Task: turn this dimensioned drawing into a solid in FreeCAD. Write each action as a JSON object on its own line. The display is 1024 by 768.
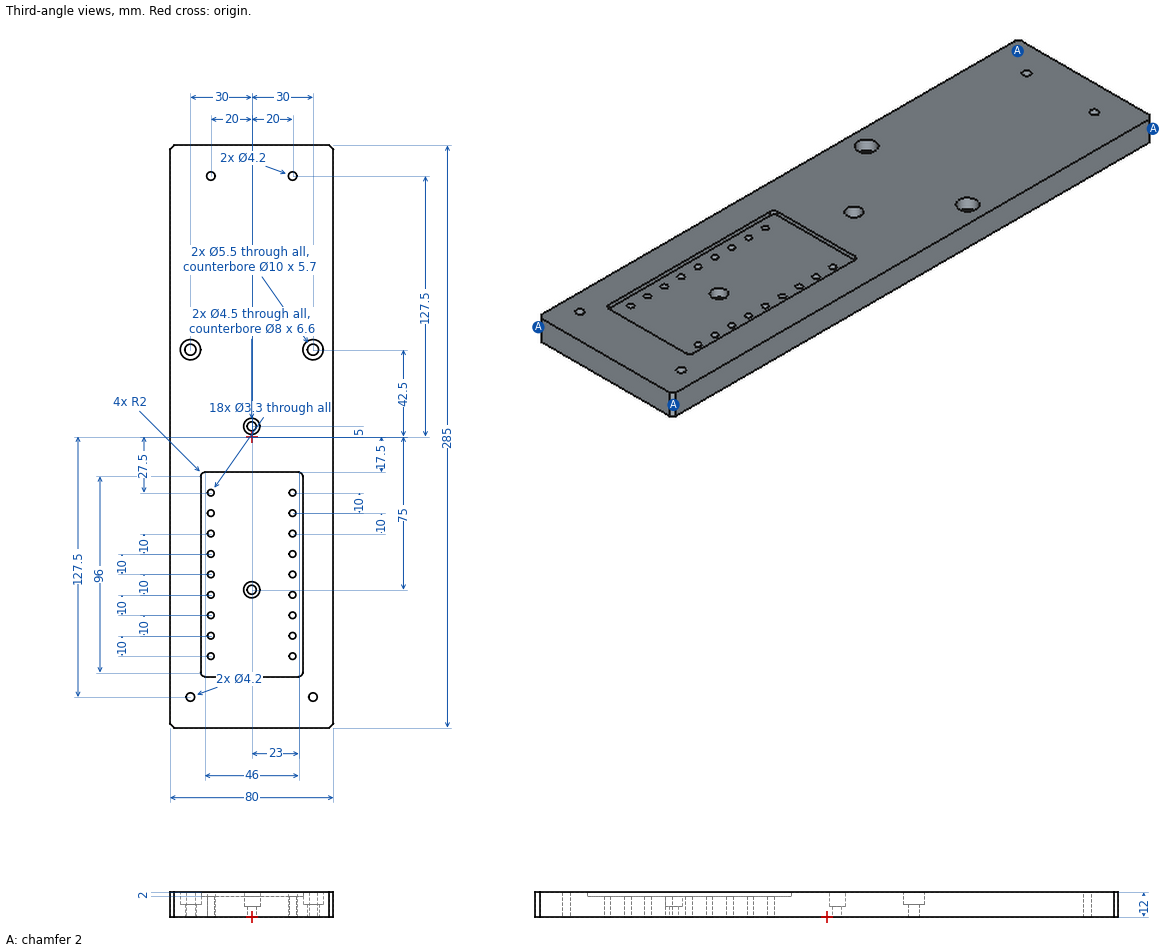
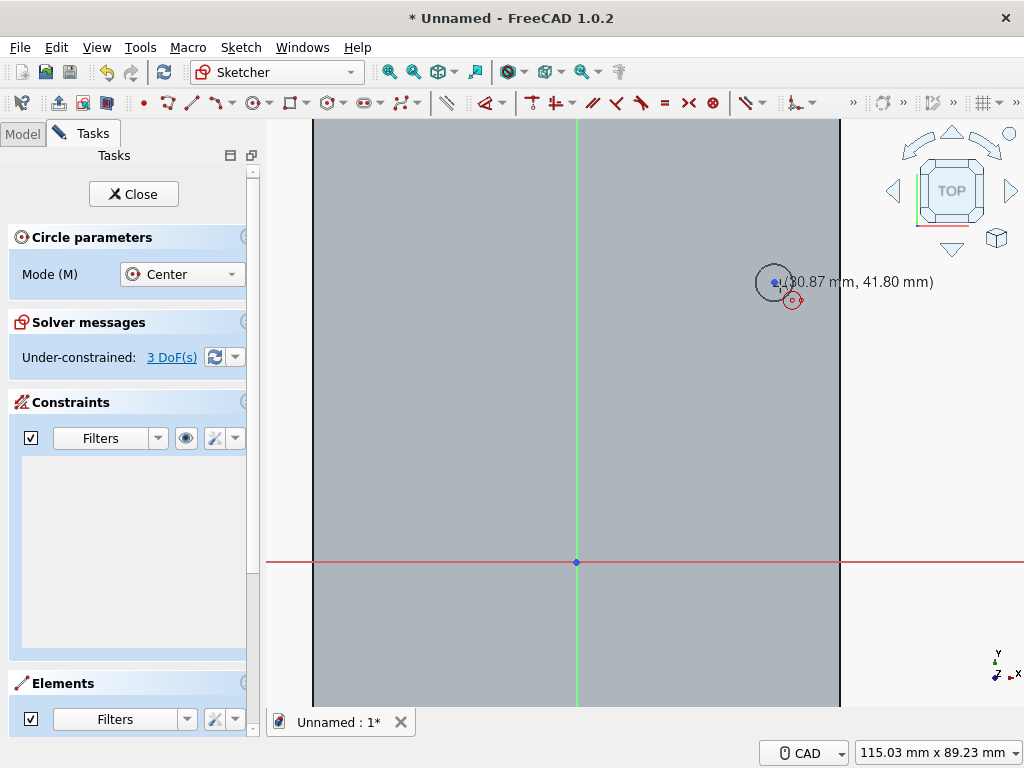
{"action": "scroll", "coordinate": [379, 282], "scroll_direction": "up", "scroll_amount": 2}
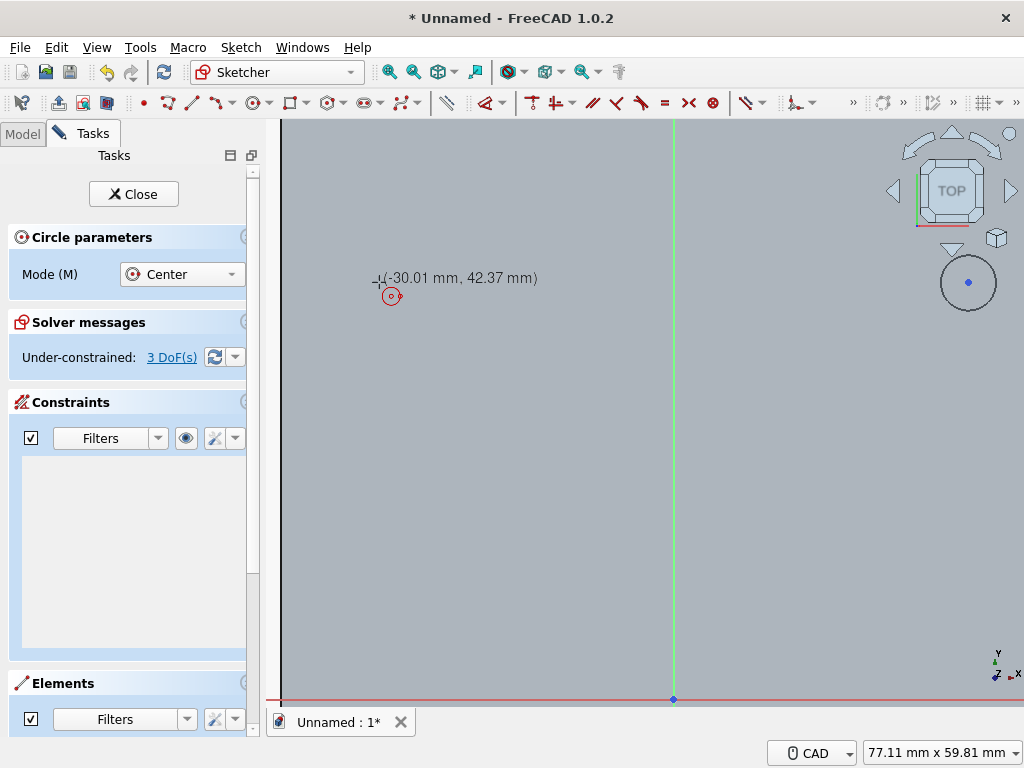
{"action": "left_click", "coordinate": [379, 282]}
{"action": "left_click", "coordinate": [398, 263]}
{"action": "key", "text": "Escape"}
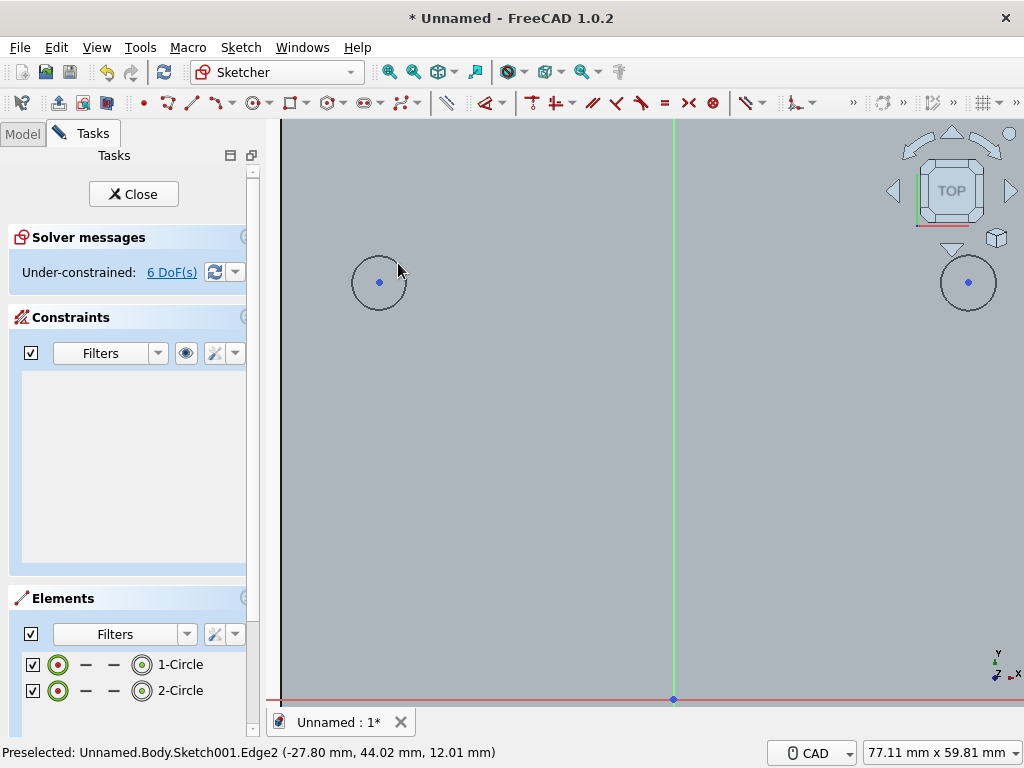
{"action": "scroll", "coordinate": [378, 282], "scroll_direction": "down", "scroll_amount": 2}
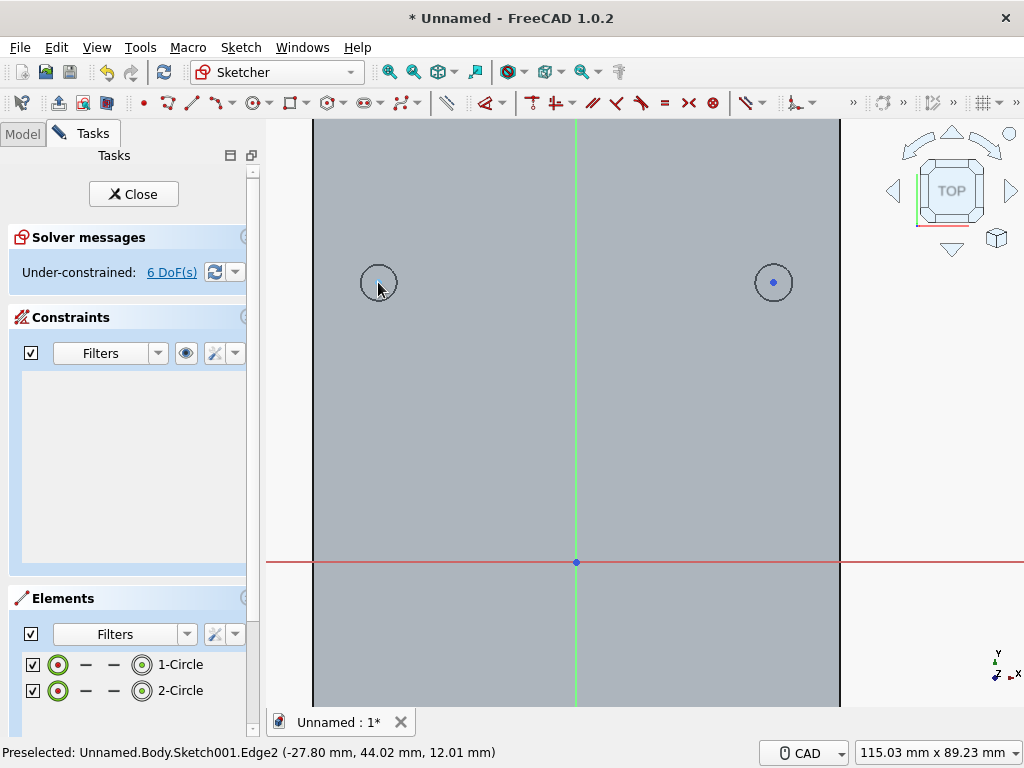
{"action": "left_click", "coordinate": [787, 270]}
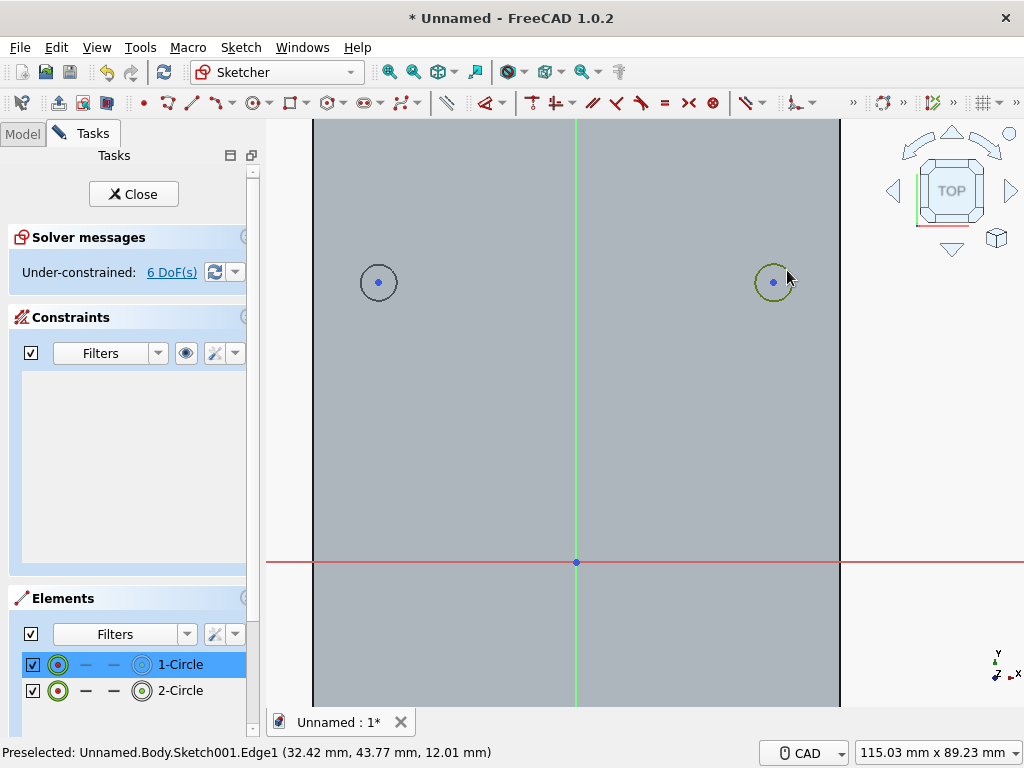
{"action": "left_click", "coordinate": [391, 270]}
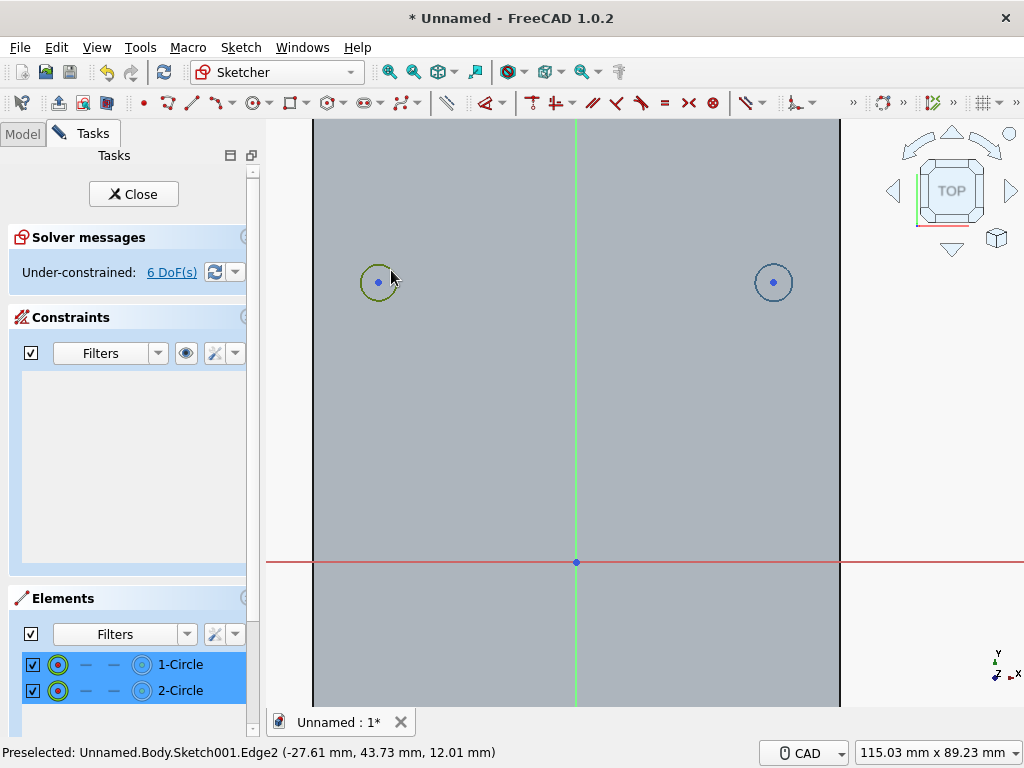
{"action": "key", "text": "e"}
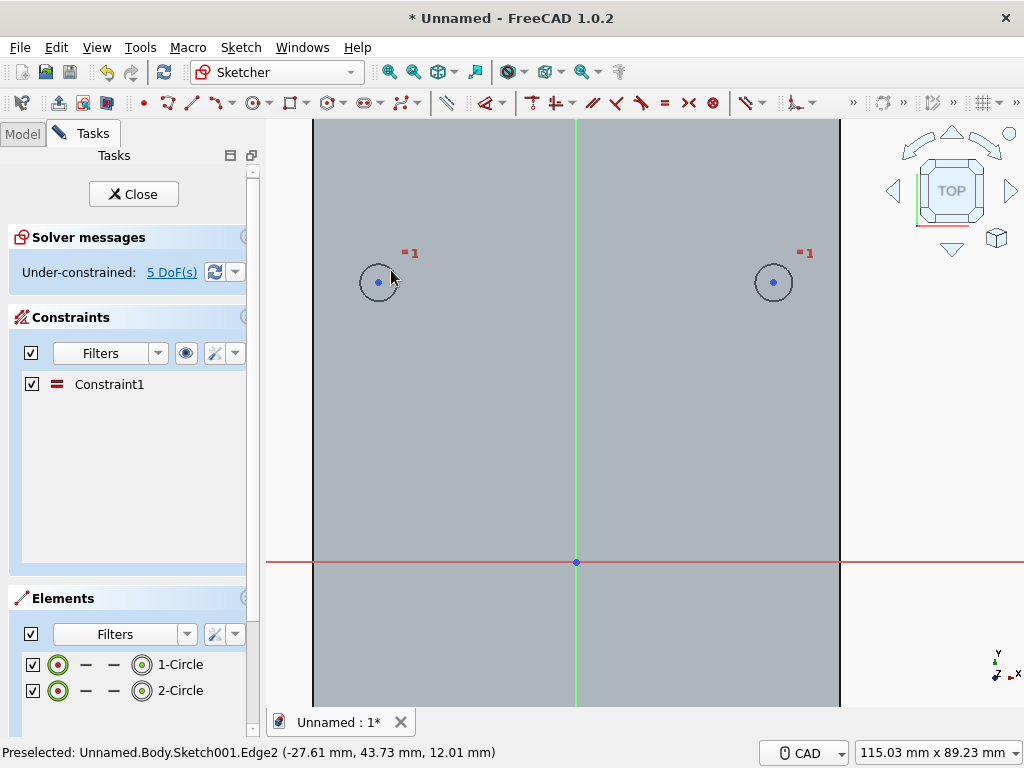
{"action": "left_click", "coordinate": [774, 283]}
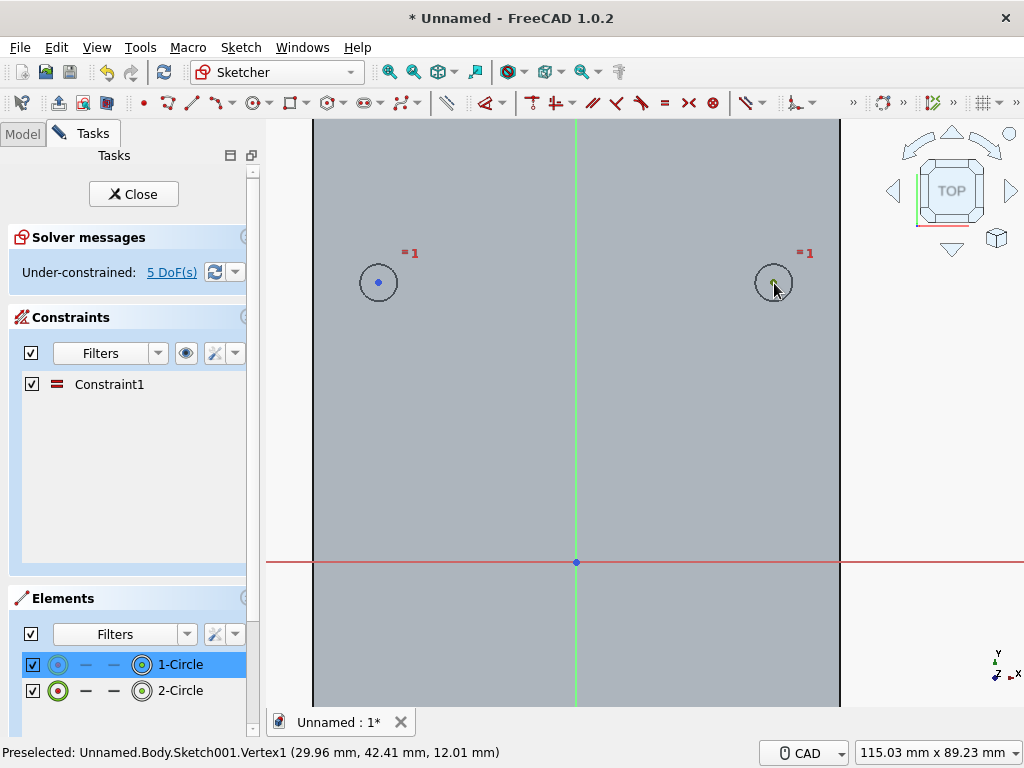
{"action": "left_click", "coordinate": [379, 283]}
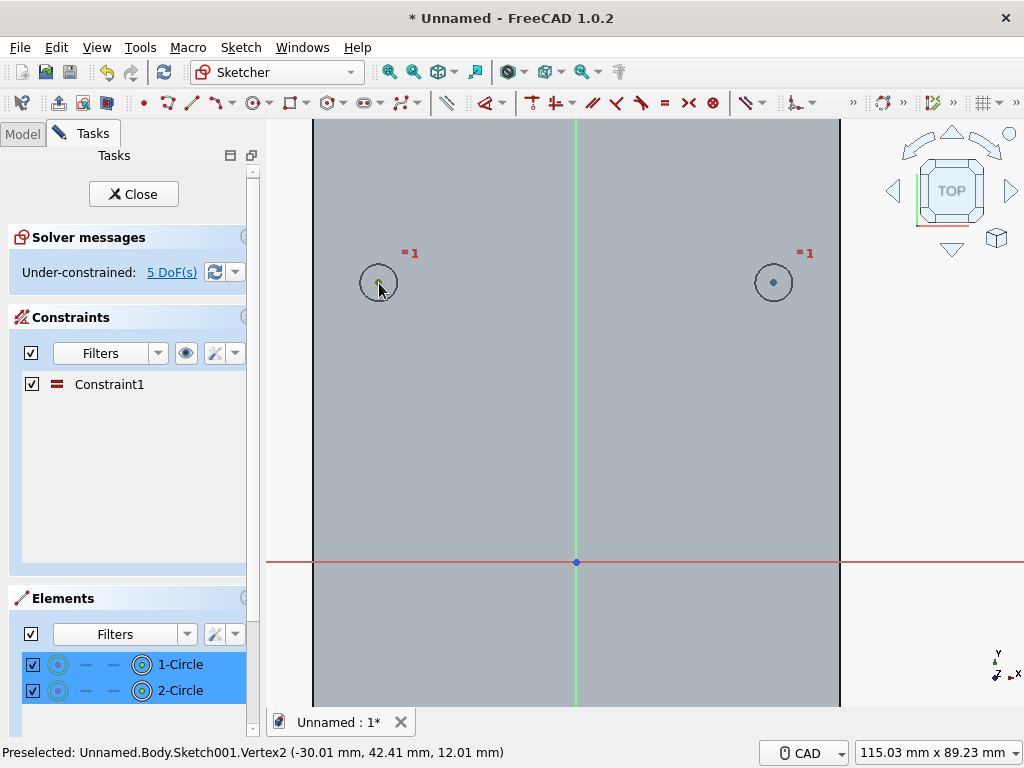
{"action": "key", "text": "h"}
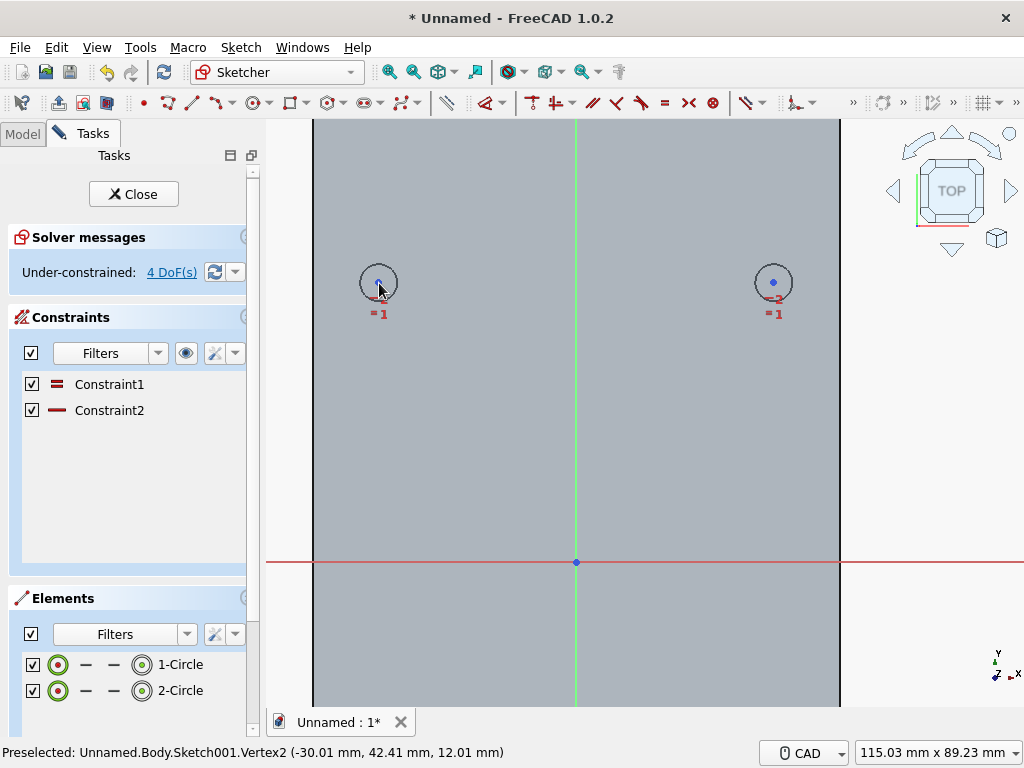
{"action": "left_click", "coordinate": [486, 104]}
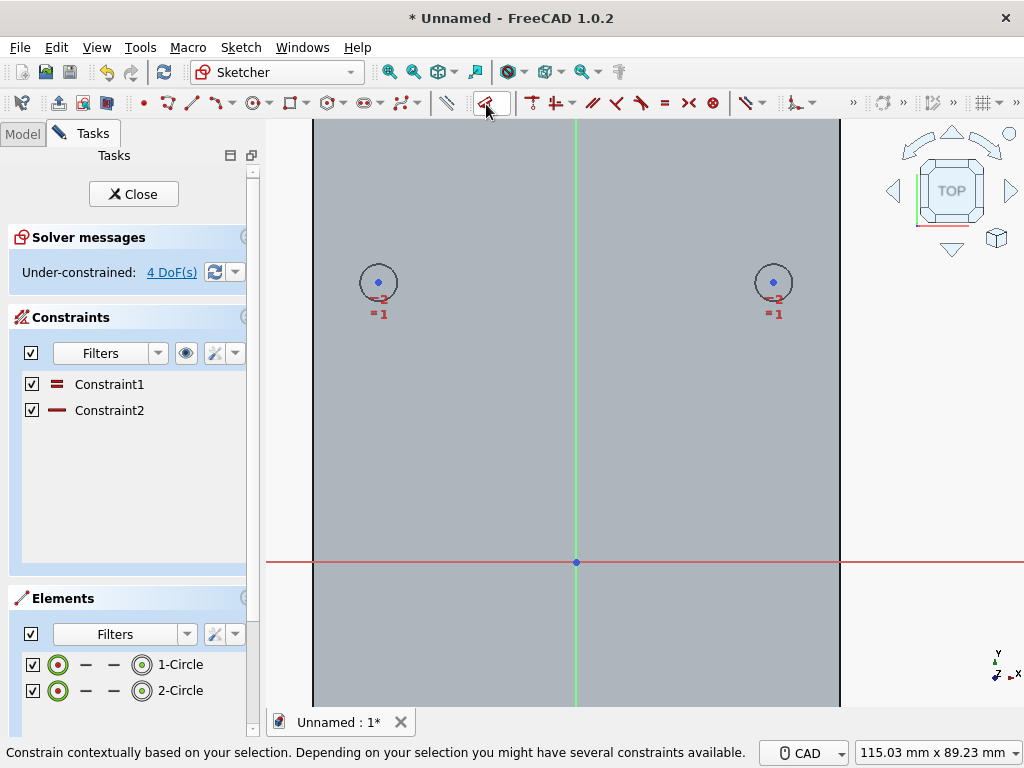
{"action": "left_click", "coordinate": [787, 270]}
{"action": "left_click", "coordinate": [810, 248]}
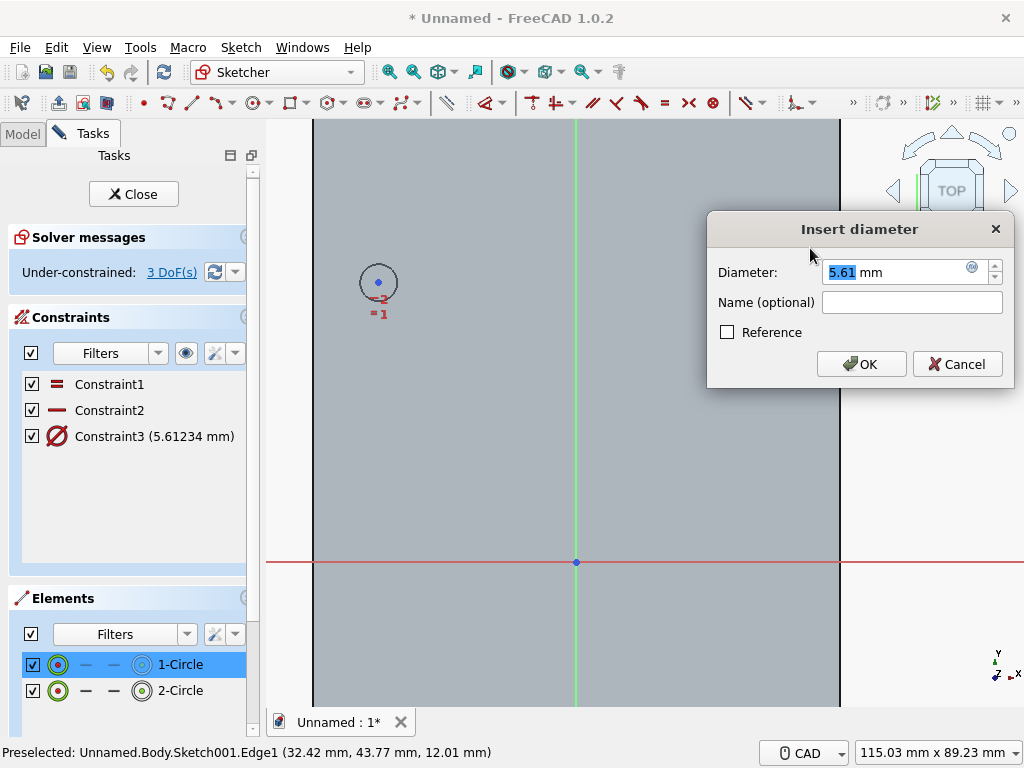
{"action": "type", "text": "5.5"}
{"action": "key", "text": "Return"}